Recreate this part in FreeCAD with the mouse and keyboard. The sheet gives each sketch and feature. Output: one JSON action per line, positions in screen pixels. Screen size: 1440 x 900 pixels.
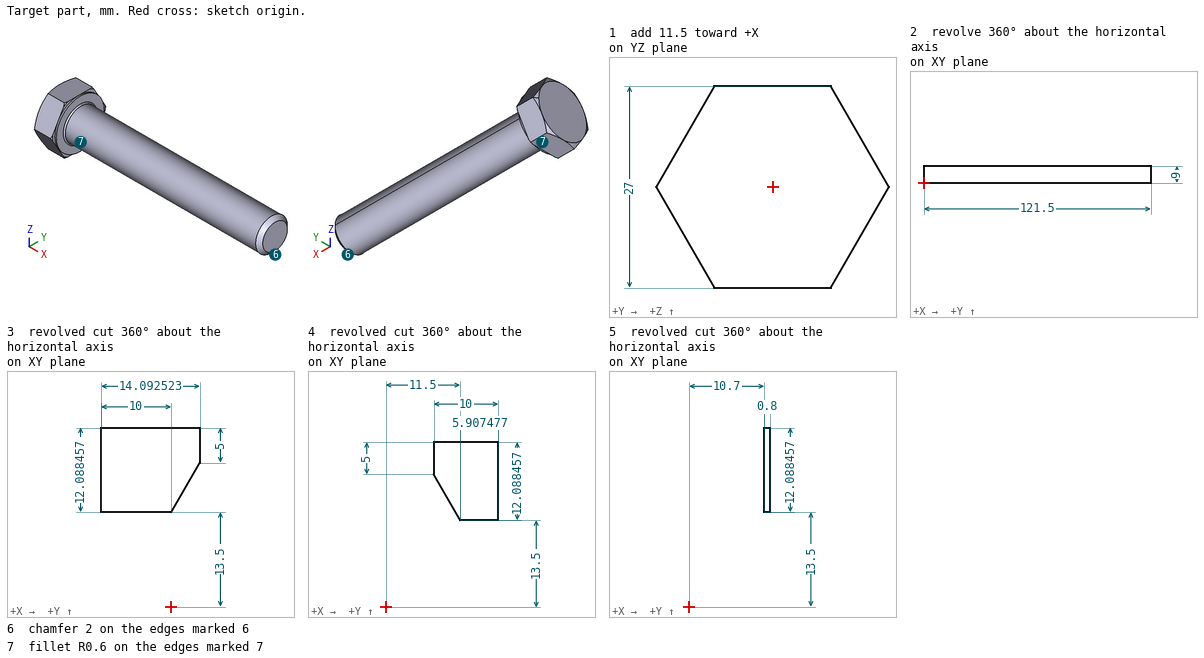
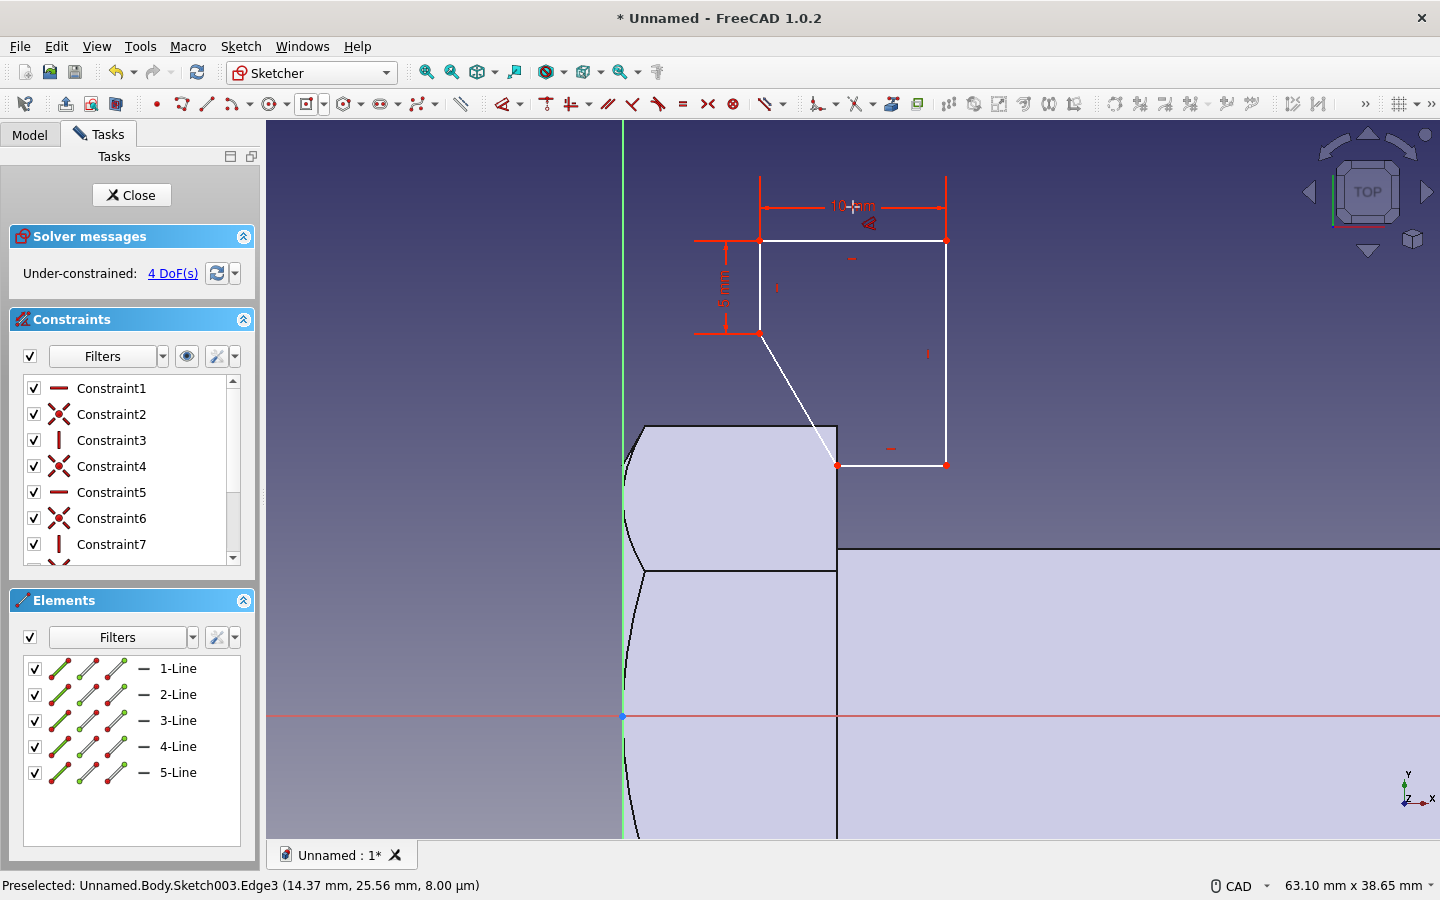
{"action": "left_click", "coordinate": [837, 466]}
{"action": "left_click", "coordinate": [730, 750]}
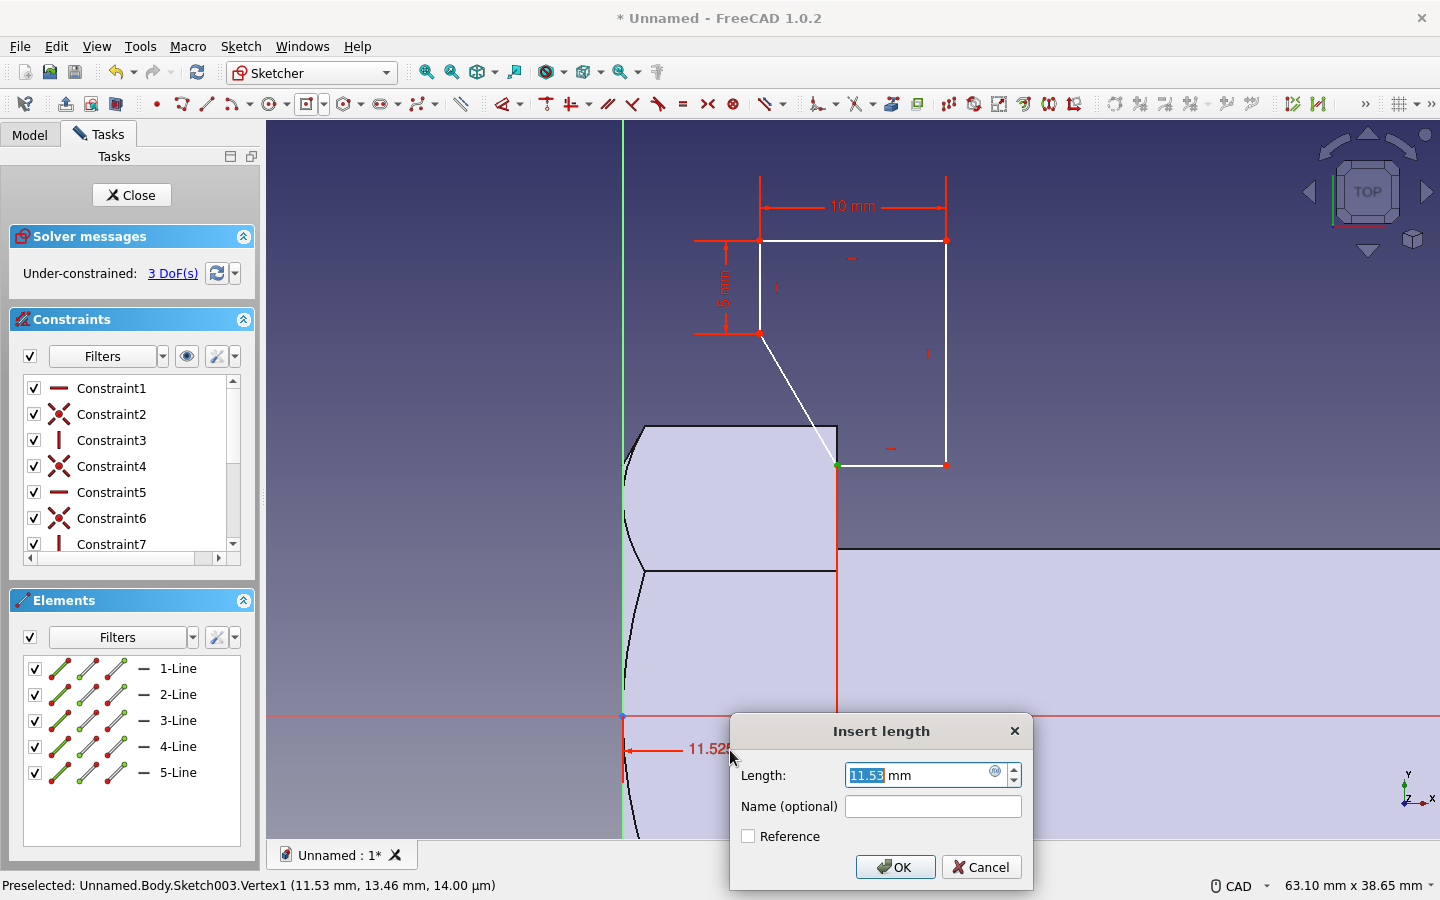
{"action": "type", "text": "11.5"}
{"action": "key", "text": "Return"}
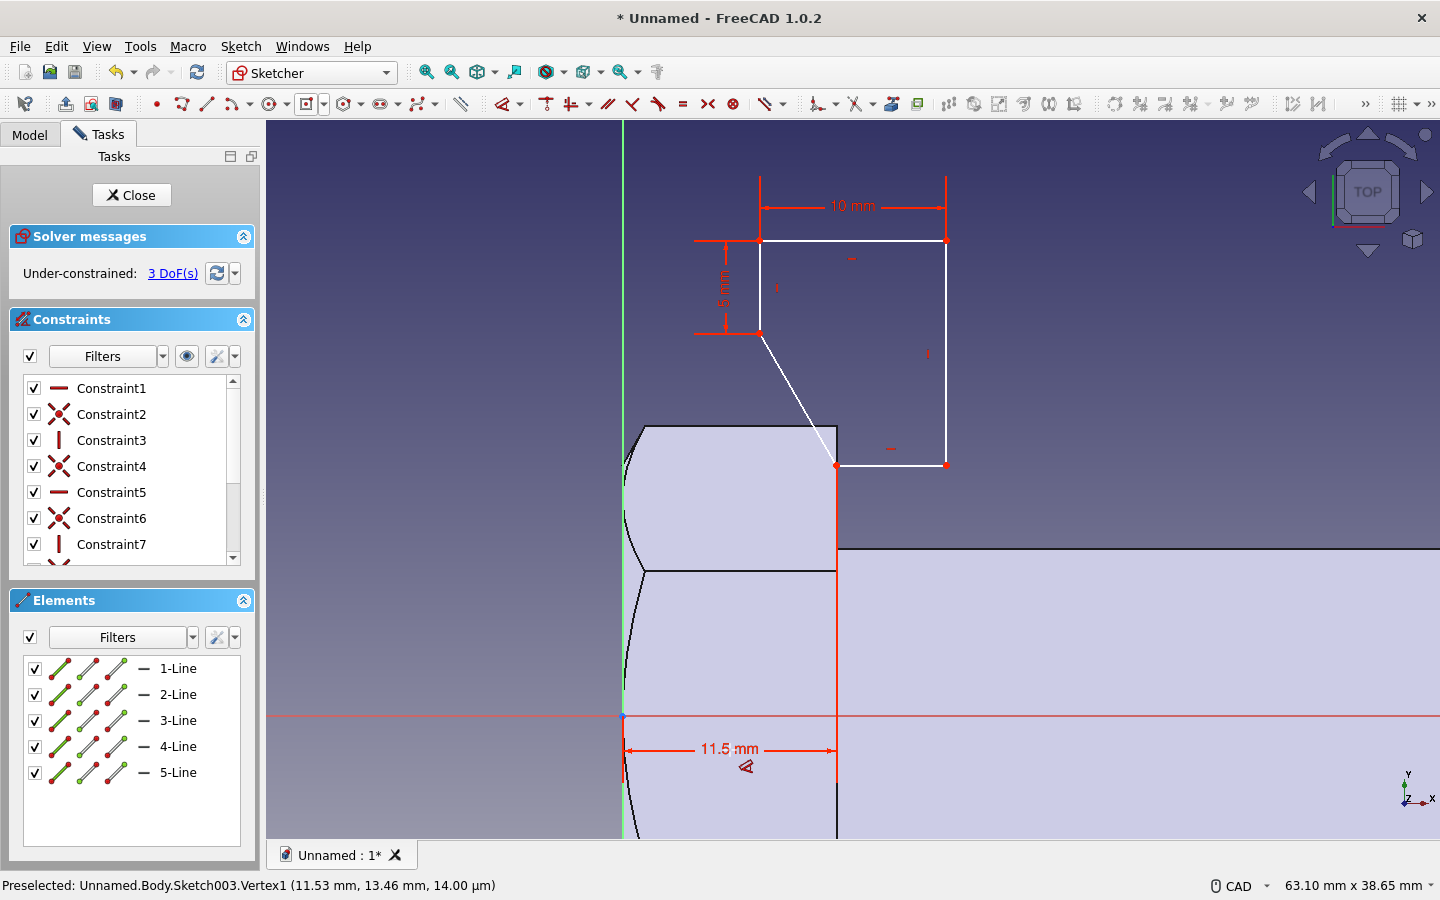
{"action": "left_click", "coordinate": [837, 466]}
{"action": "left_click", "coordinate": [589, 591]}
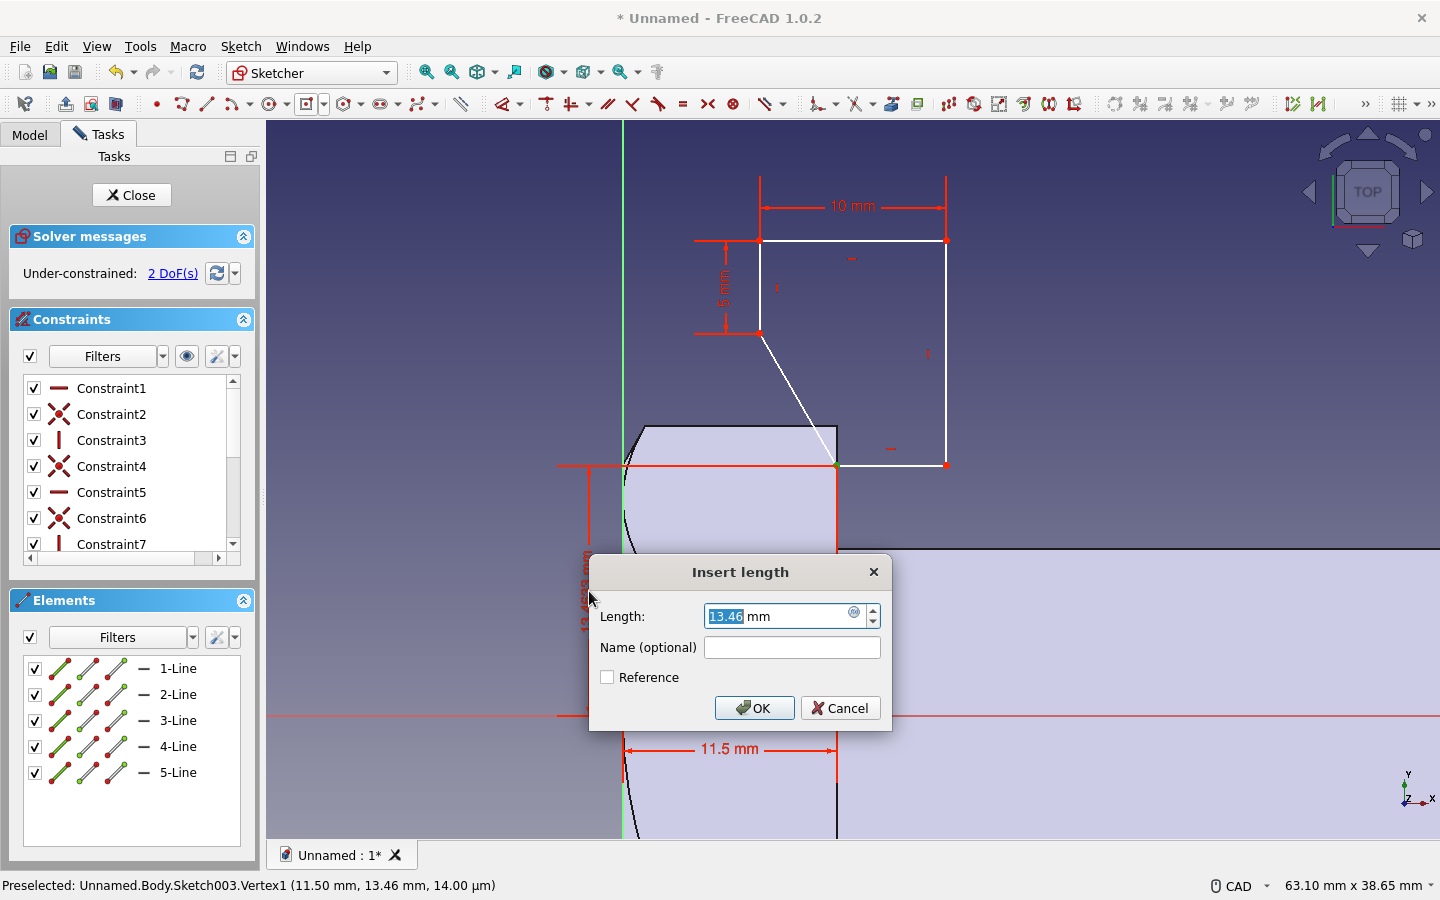
{"action": "type", "text": "13.5"}
{"action": "key", "text": "Return"}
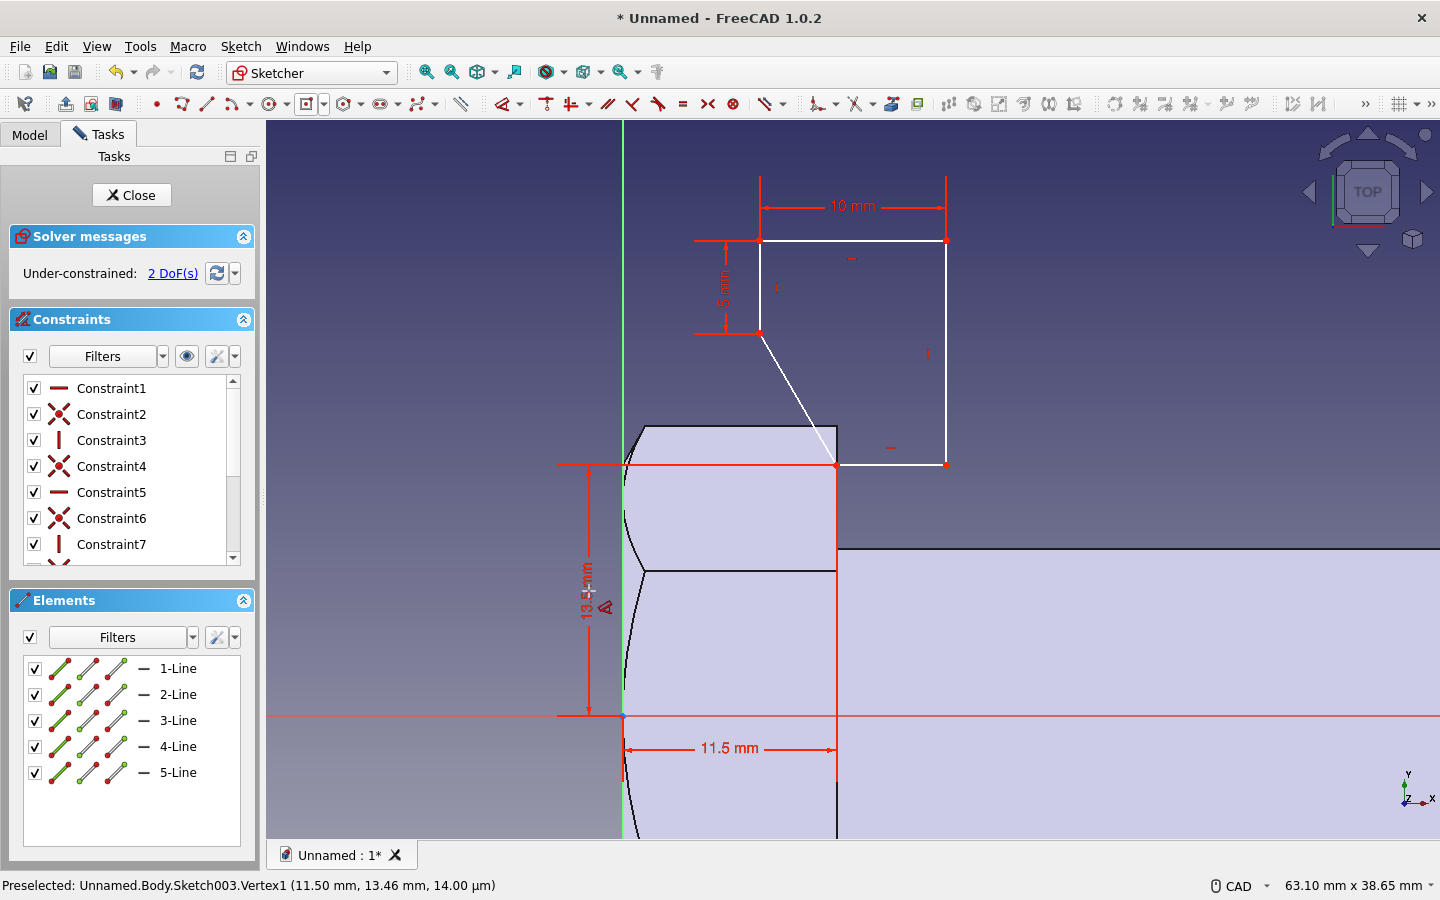
{"action": "left_click", "coordinate": [869, 465]}
{"action": "left_click", "coordinate": [891, 431]}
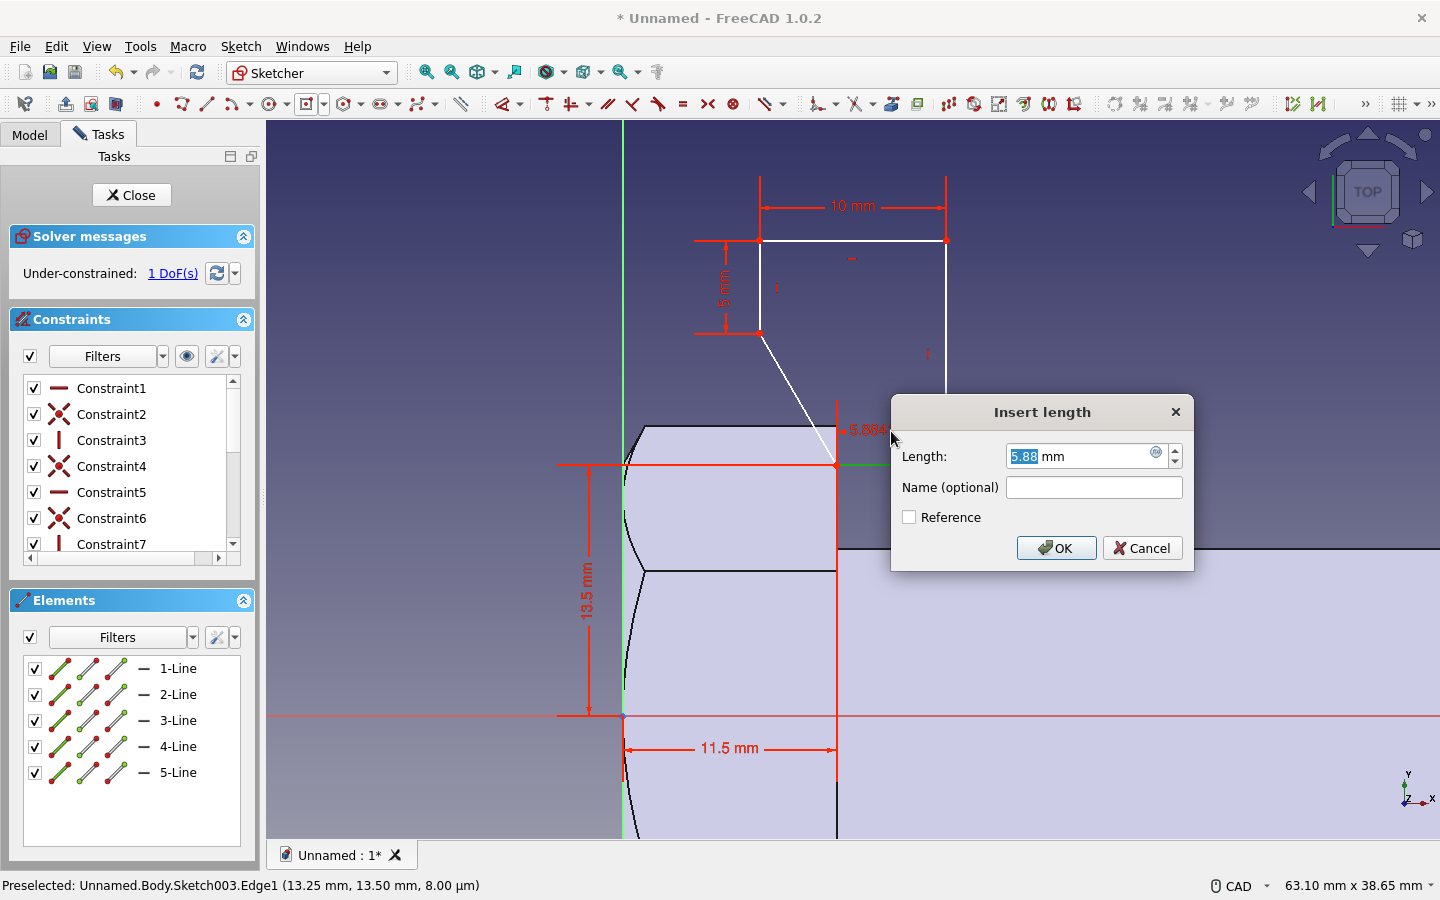
{"action": "type", "text": "5.907477"}
{"action": "key", "text": "Return"}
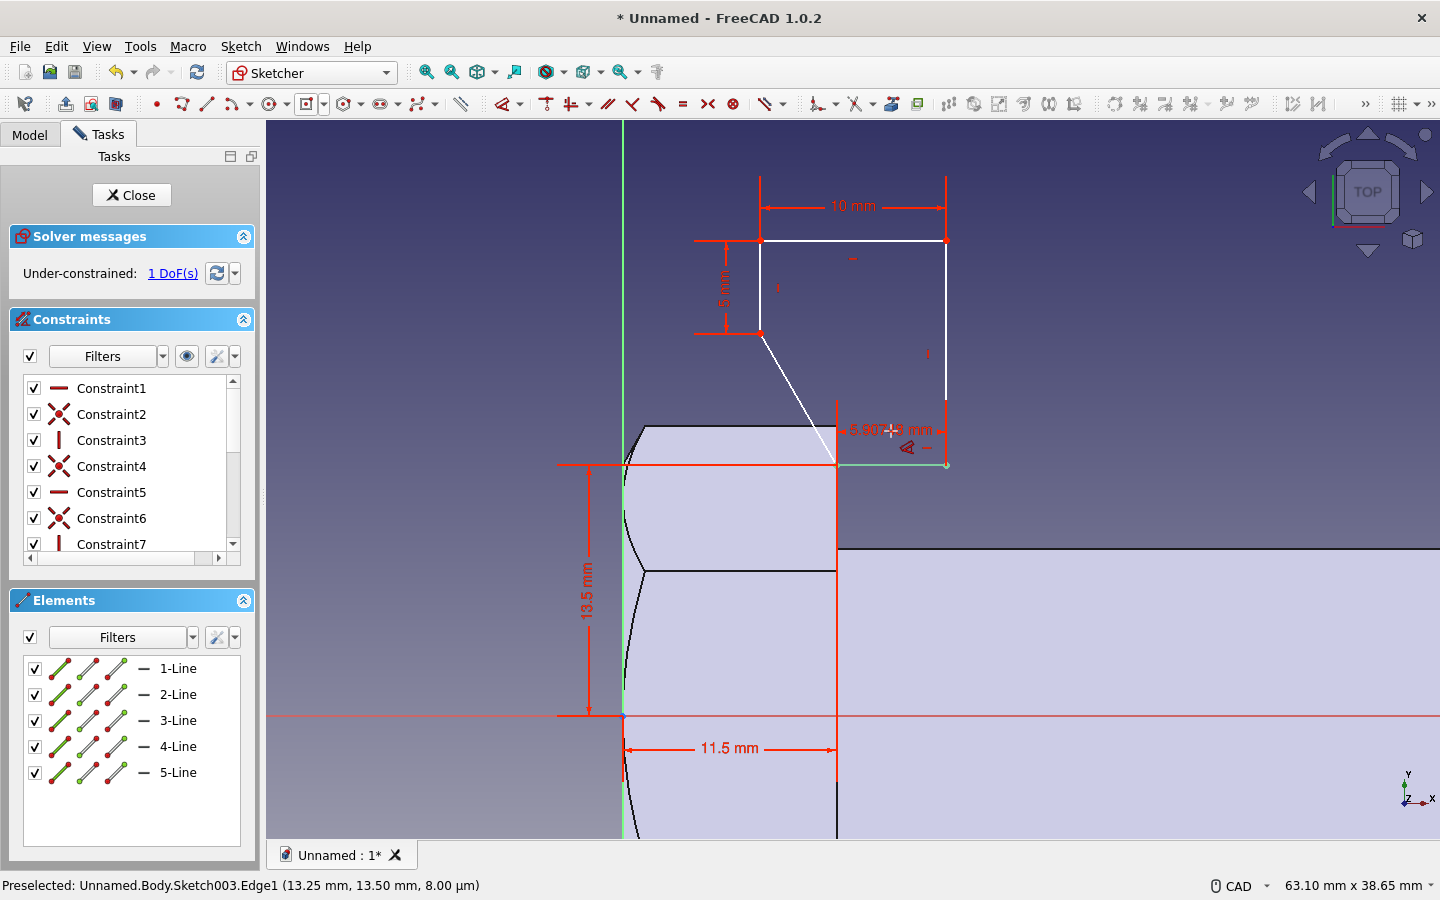
{"action": "left_click", "coordinate": [946, 398]}
{"action": "left_click", "coordinate": [980, 353]}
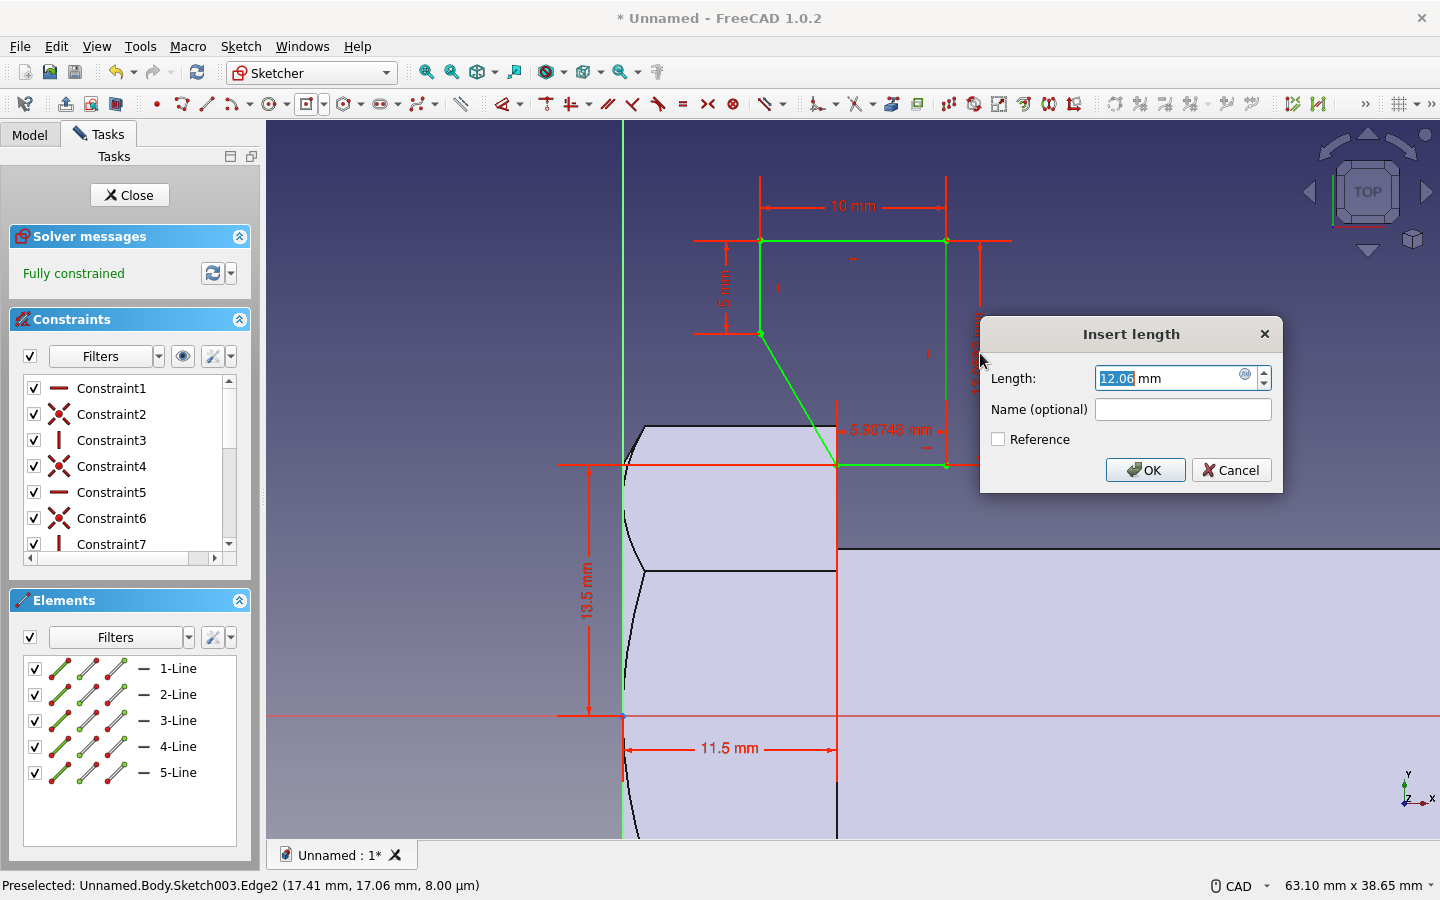
{"action": "type", "text": "12.088457"}
{"action": "key", "text": "Return"}
{"action": "key", "text": "Escape"}